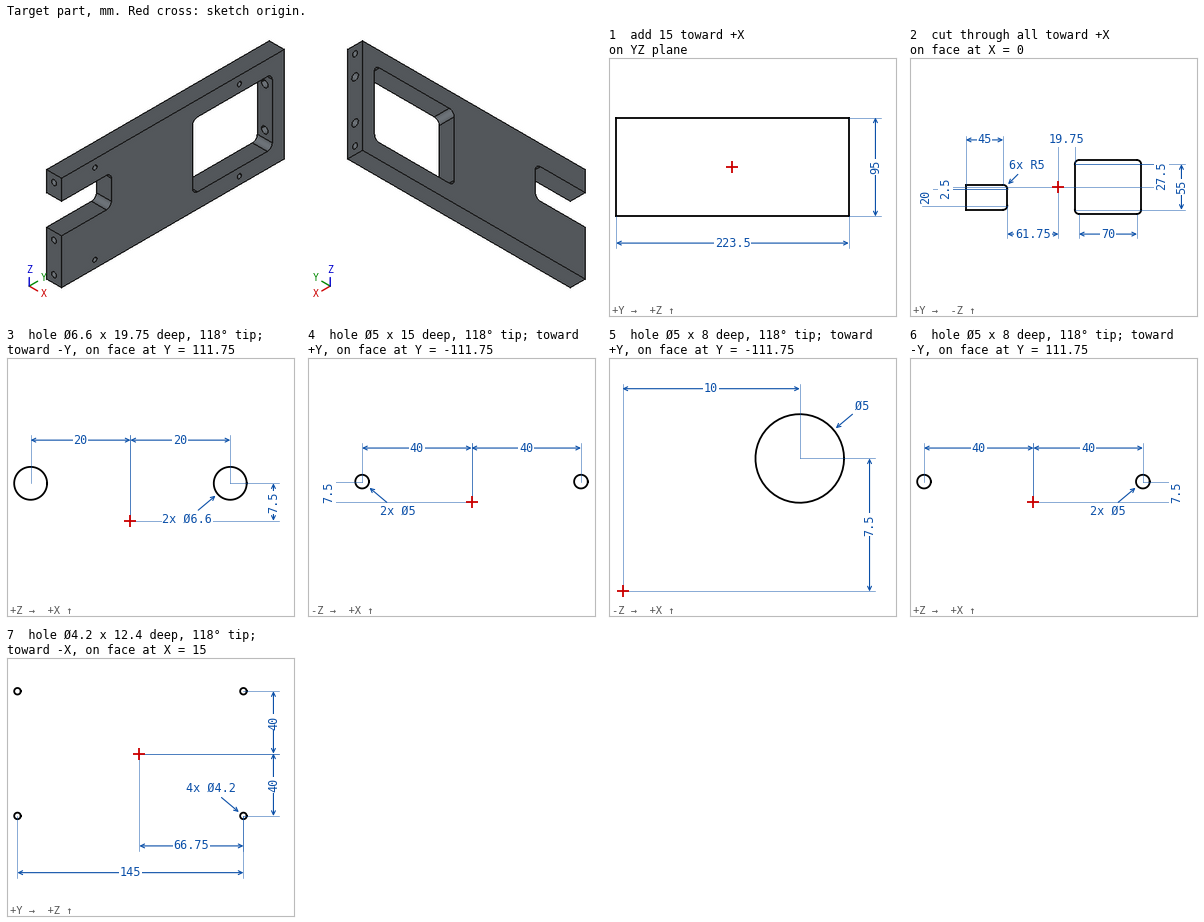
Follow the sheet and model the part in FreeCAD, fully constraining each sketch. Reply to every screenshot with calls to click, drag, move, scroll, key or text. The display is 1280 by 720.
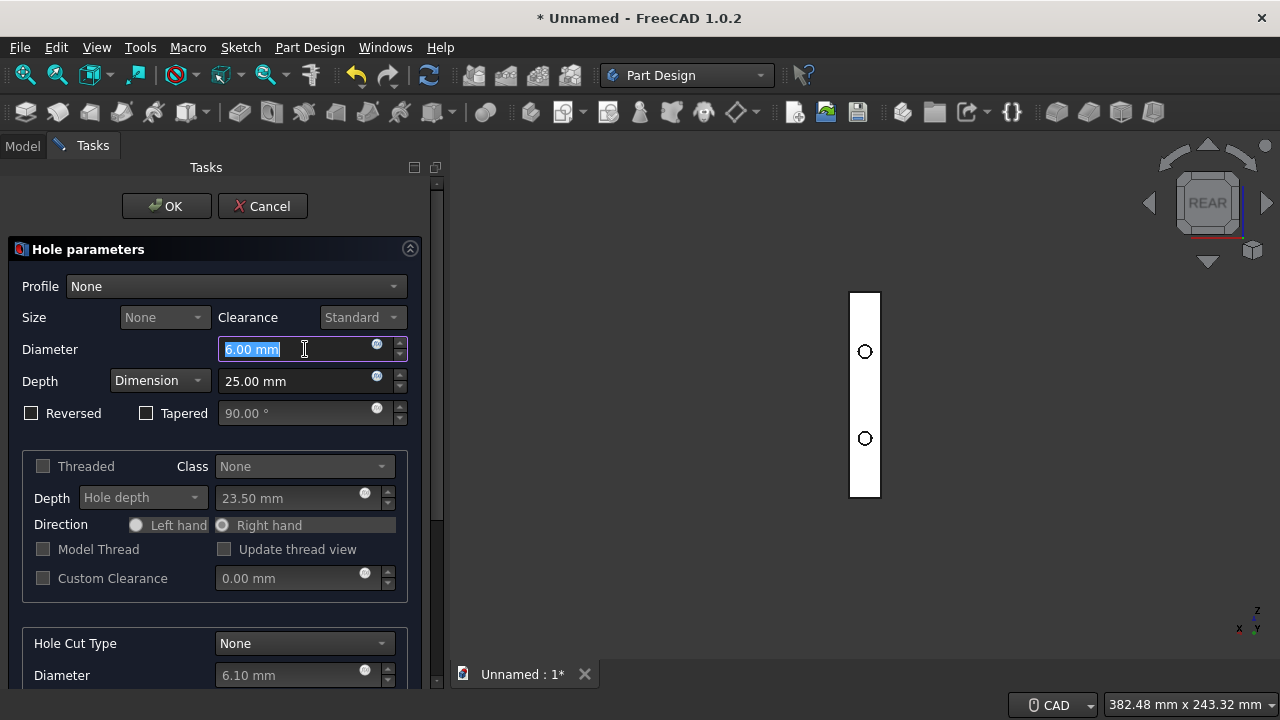
text(6.6)
key(Tab)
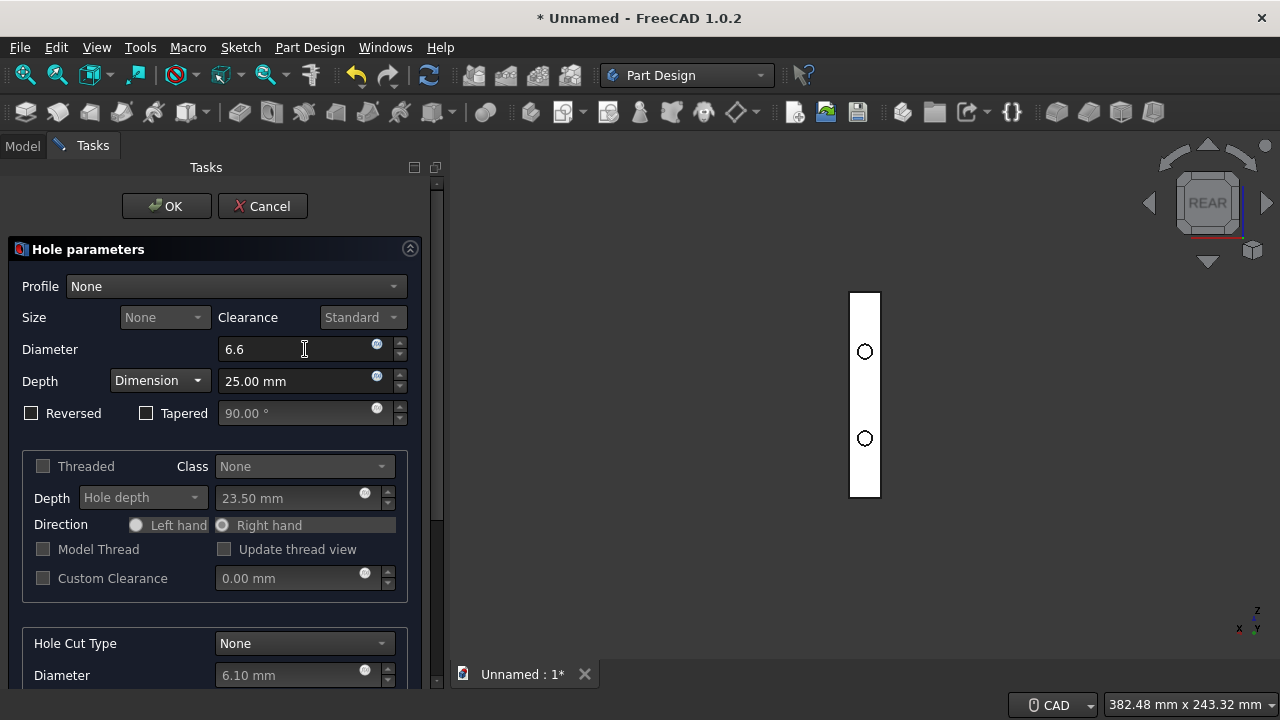
triple_click(305, 381)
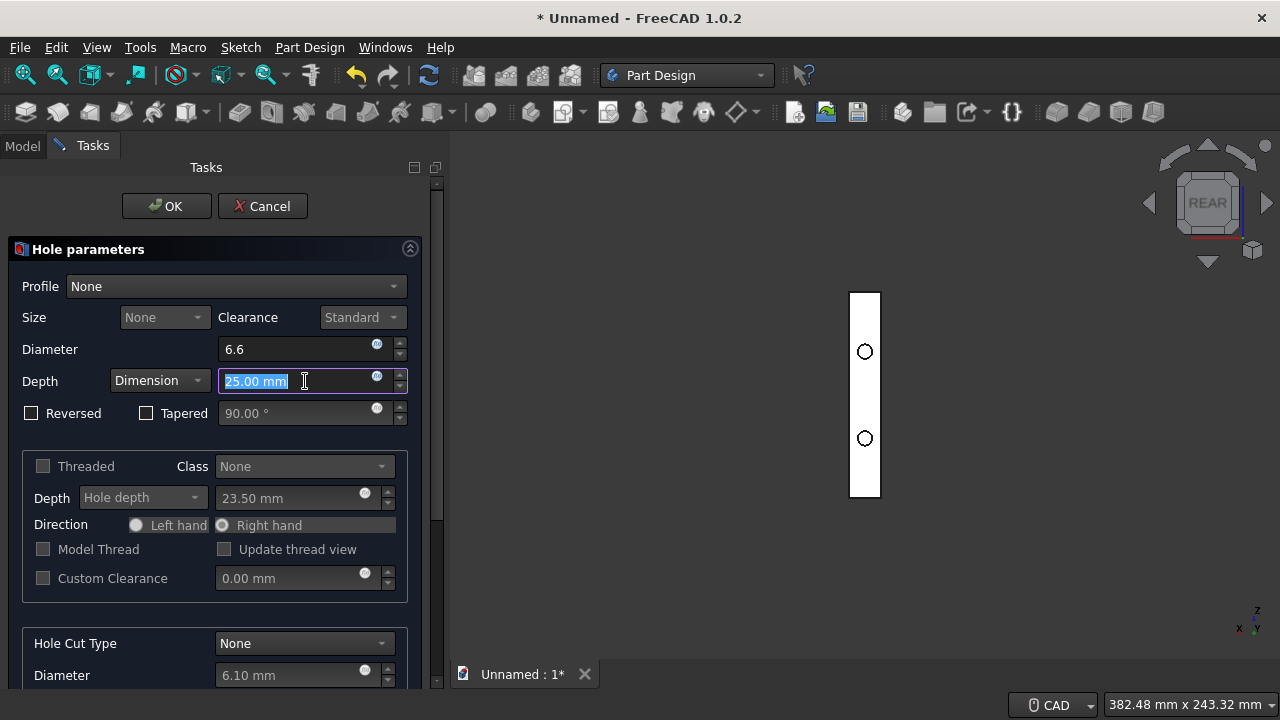
text(19.75)
key(Tab)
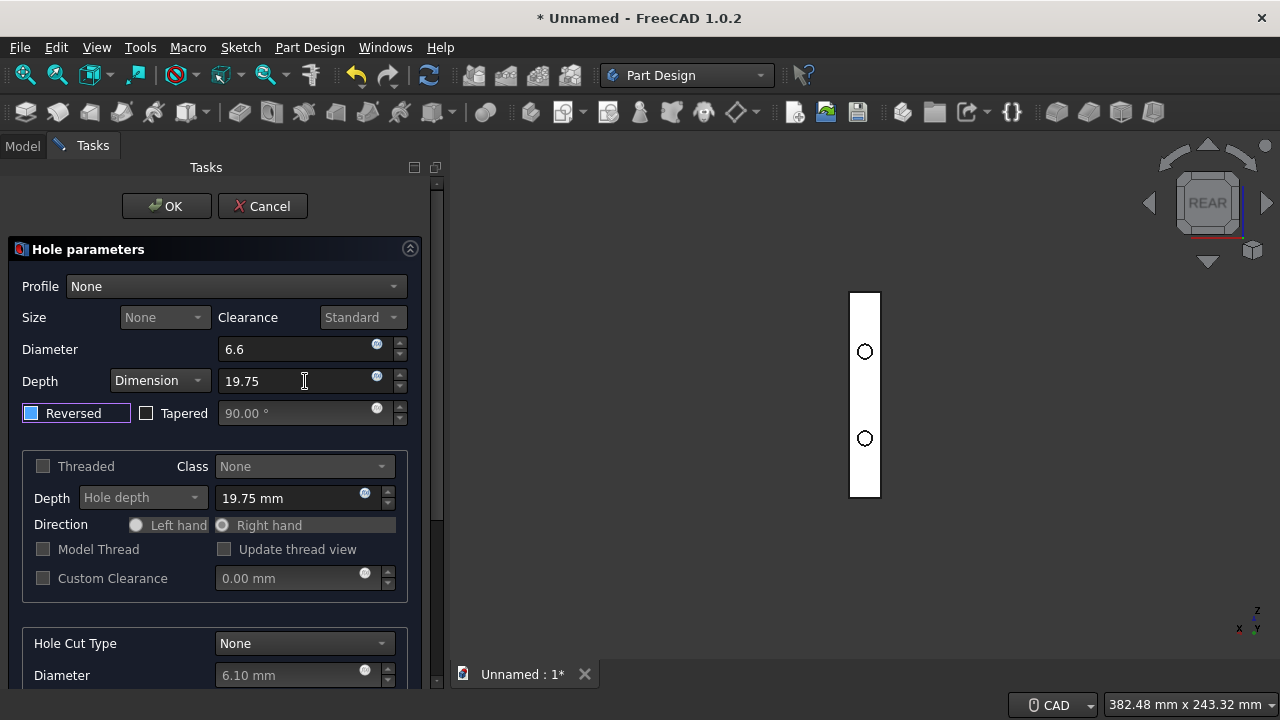
click(167, 206)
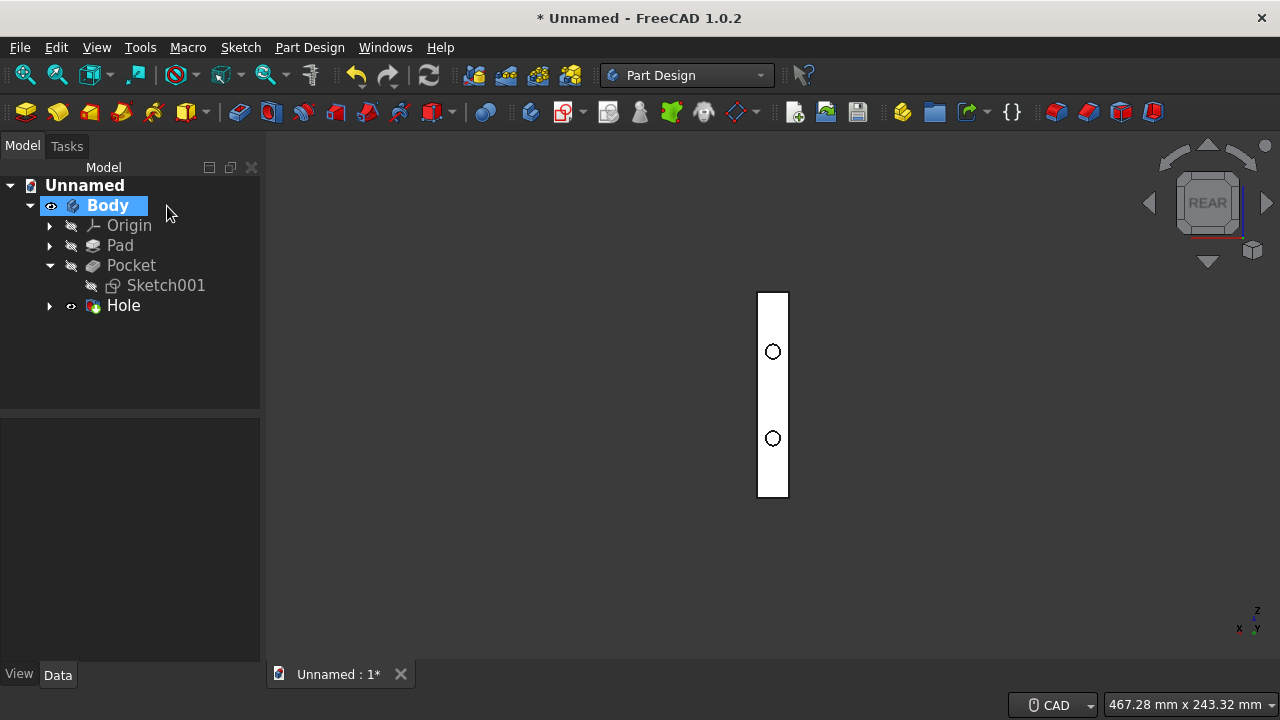
click(26, 76)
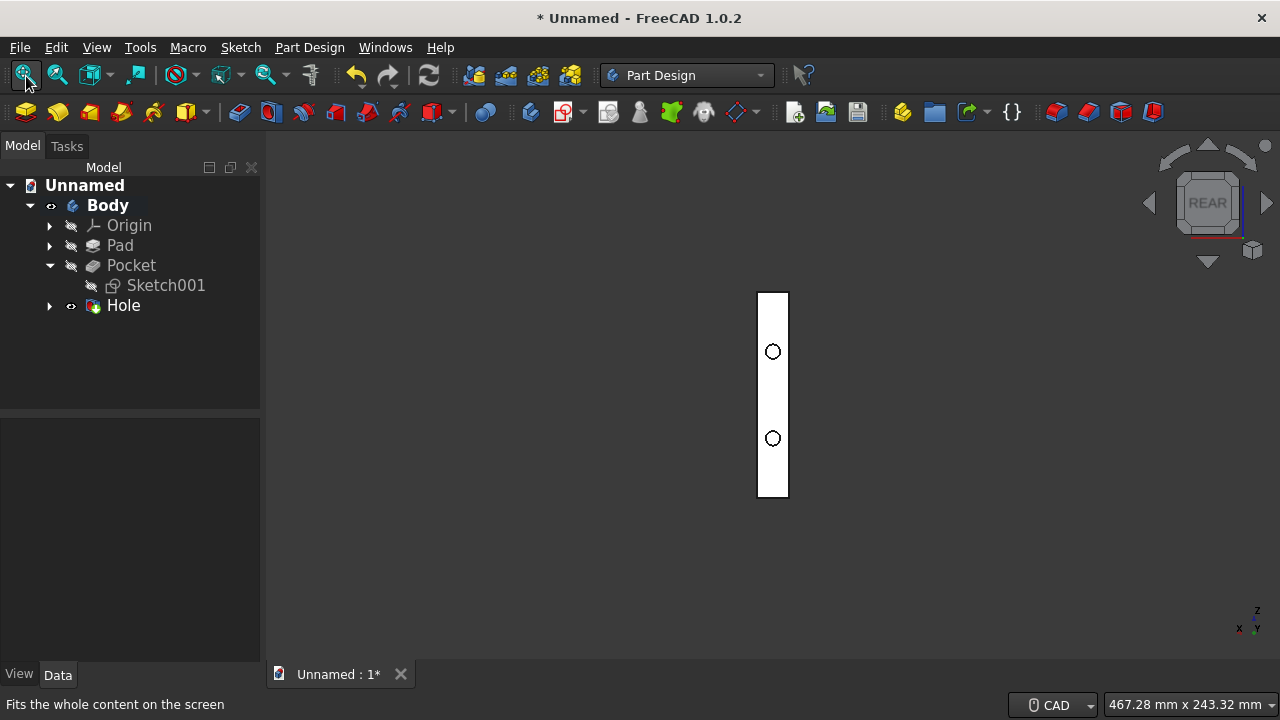
key(0)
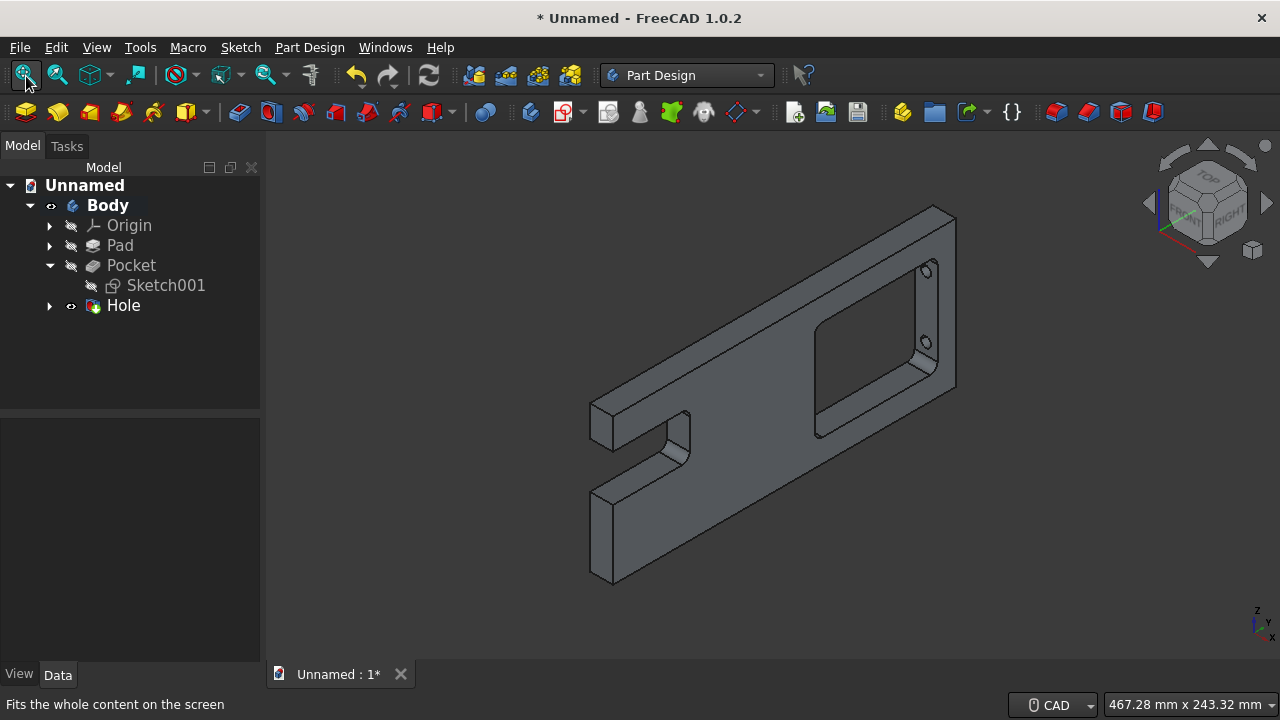
click(602, 560)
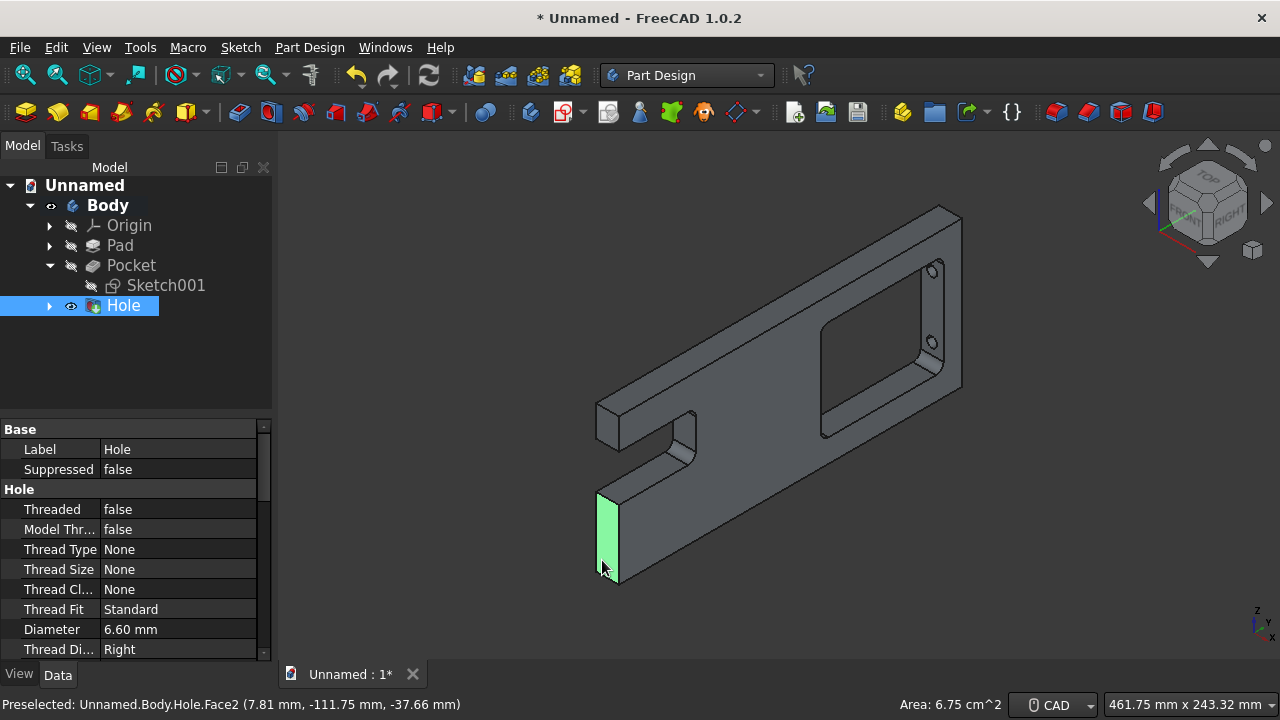
click(564, 112)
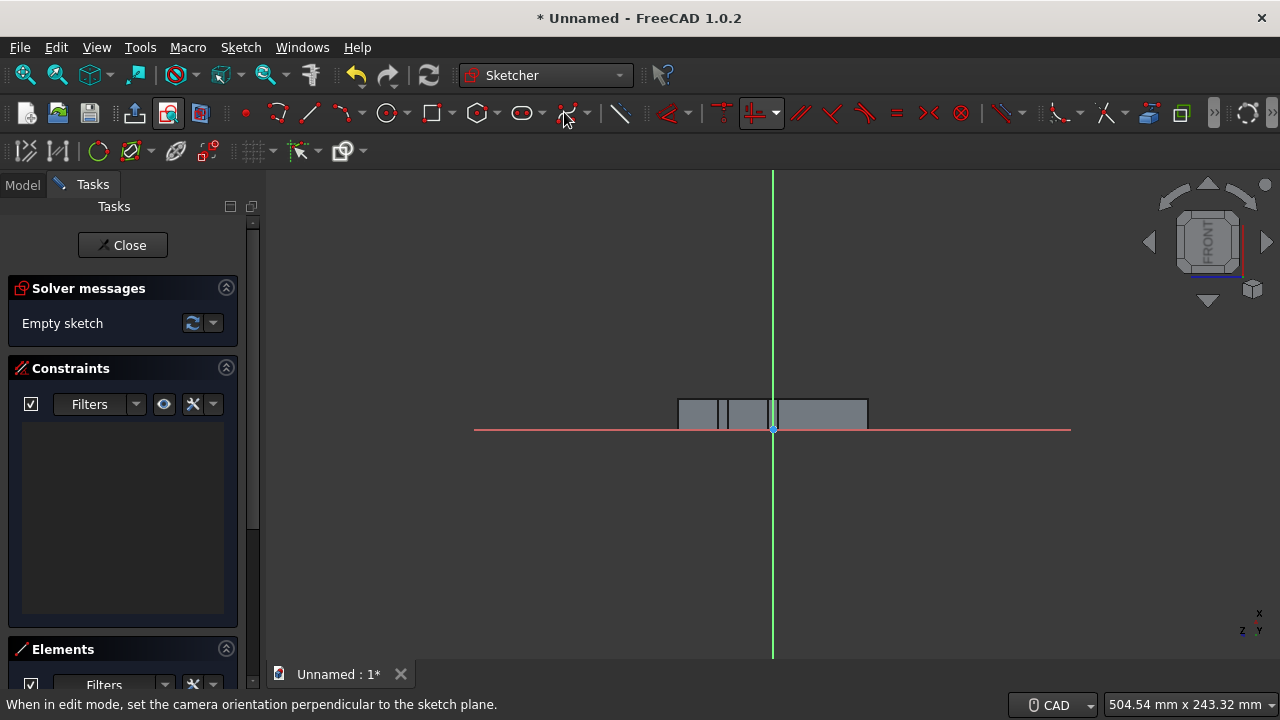
scroll(803, 422, up, 6)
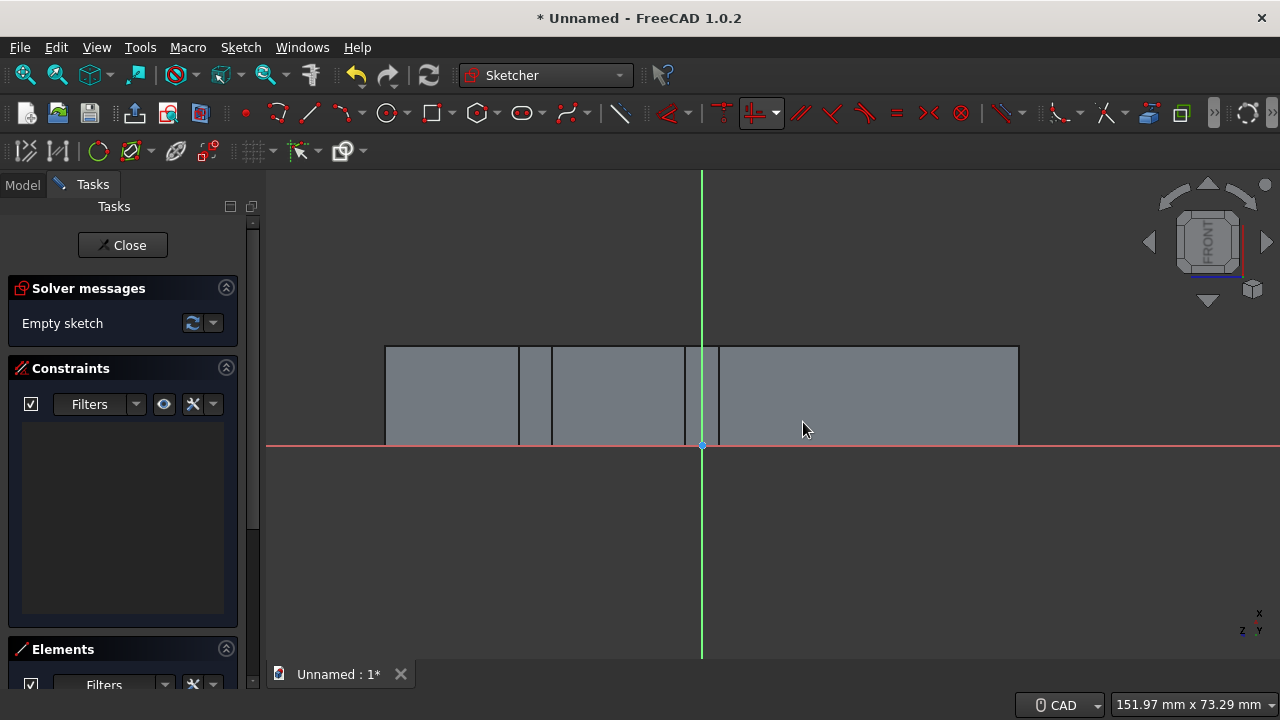
click(388, 114)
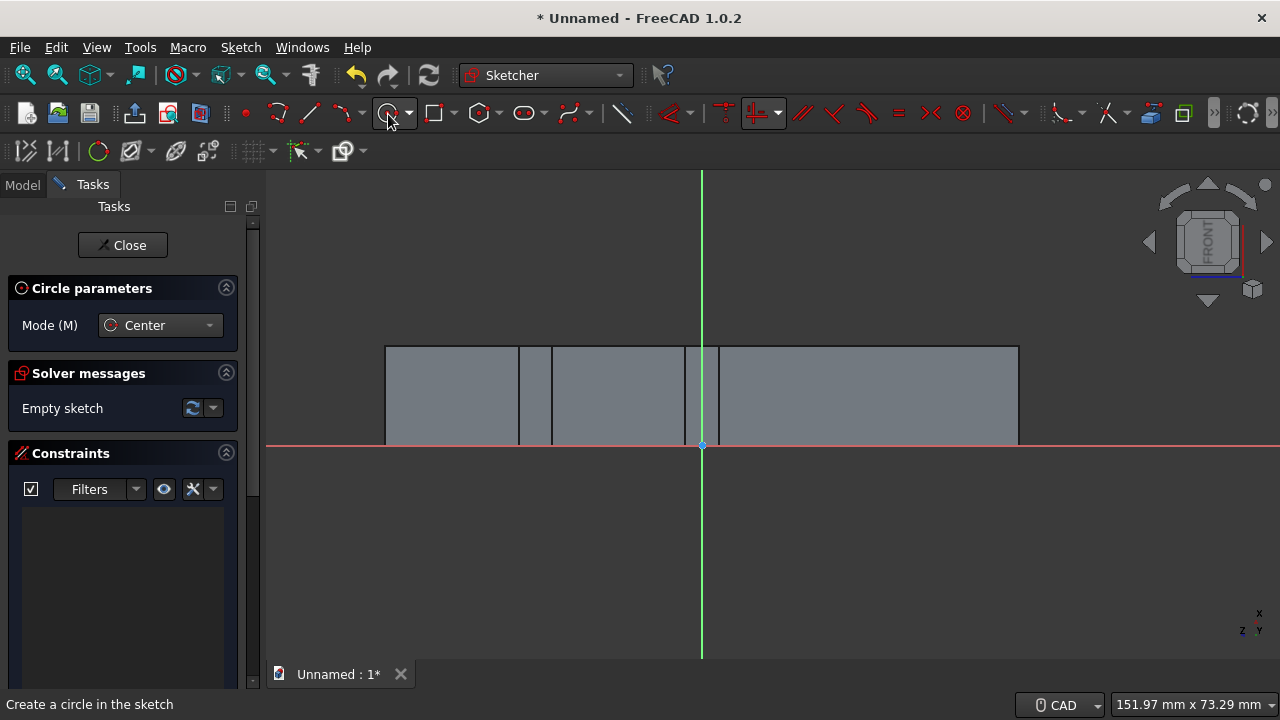
scroll(435, 396, up, 2)